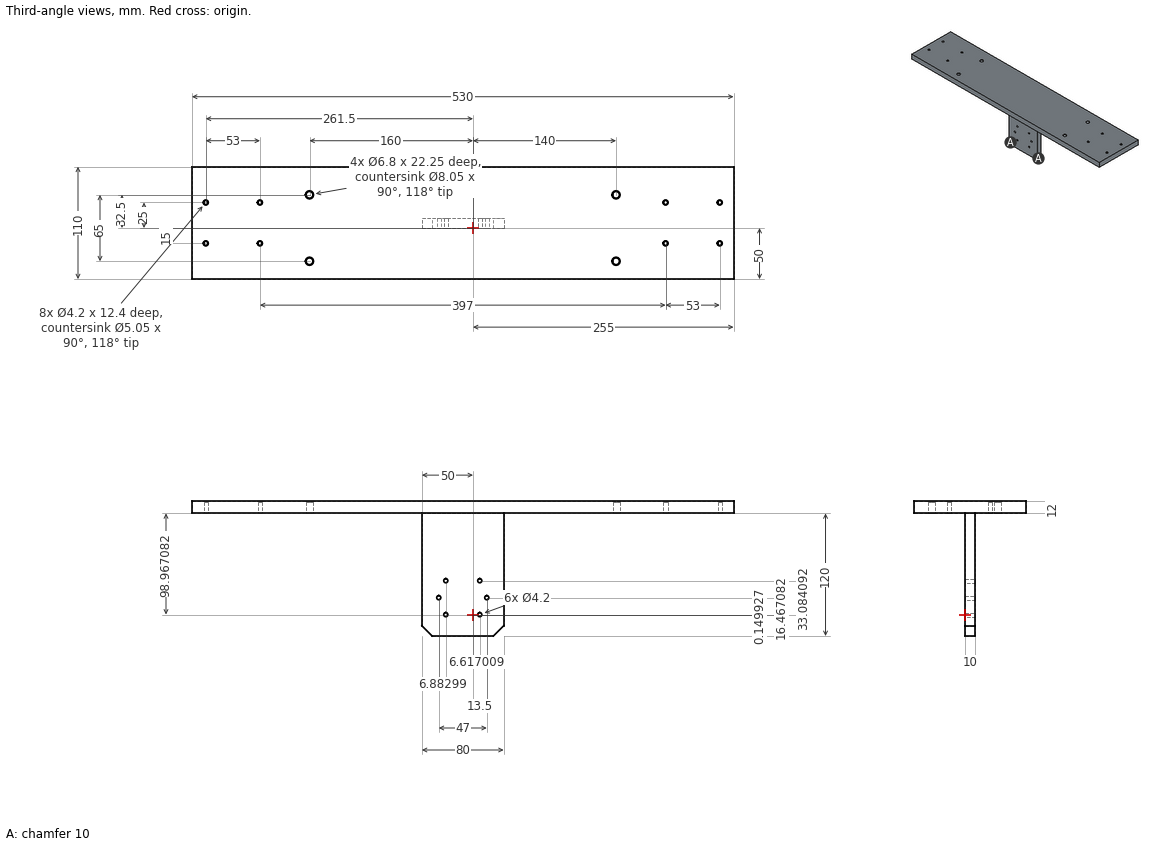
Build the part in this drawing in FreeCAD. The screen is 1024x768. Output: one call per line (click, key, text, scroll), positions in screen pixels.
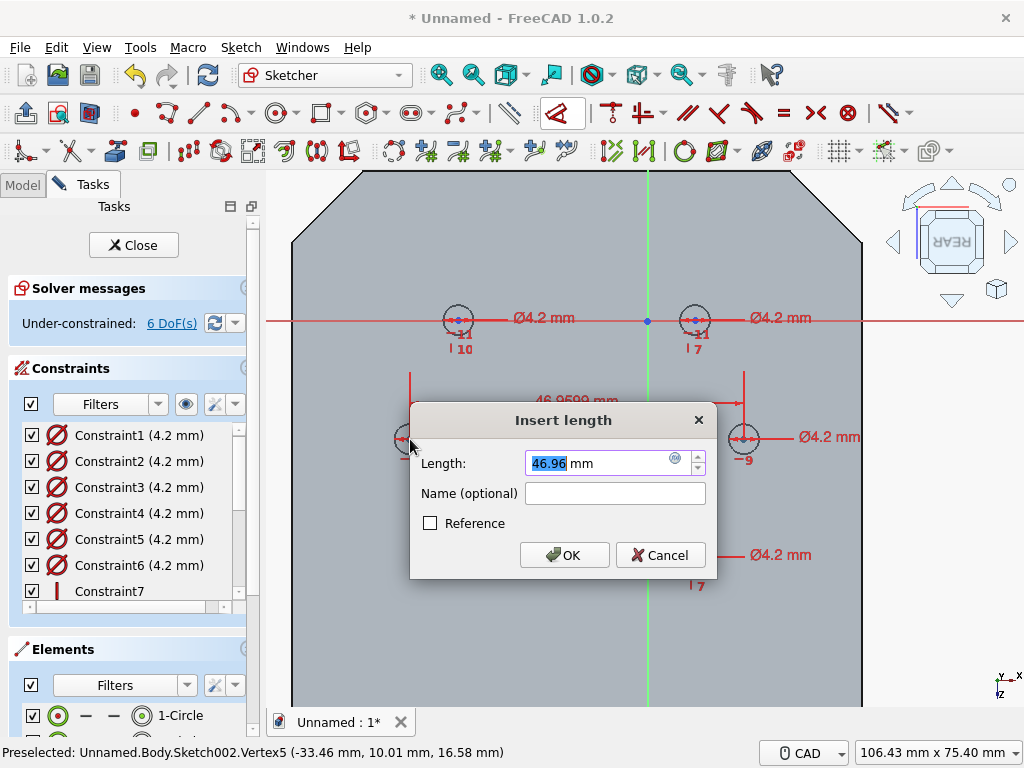
text(47)
key(Return)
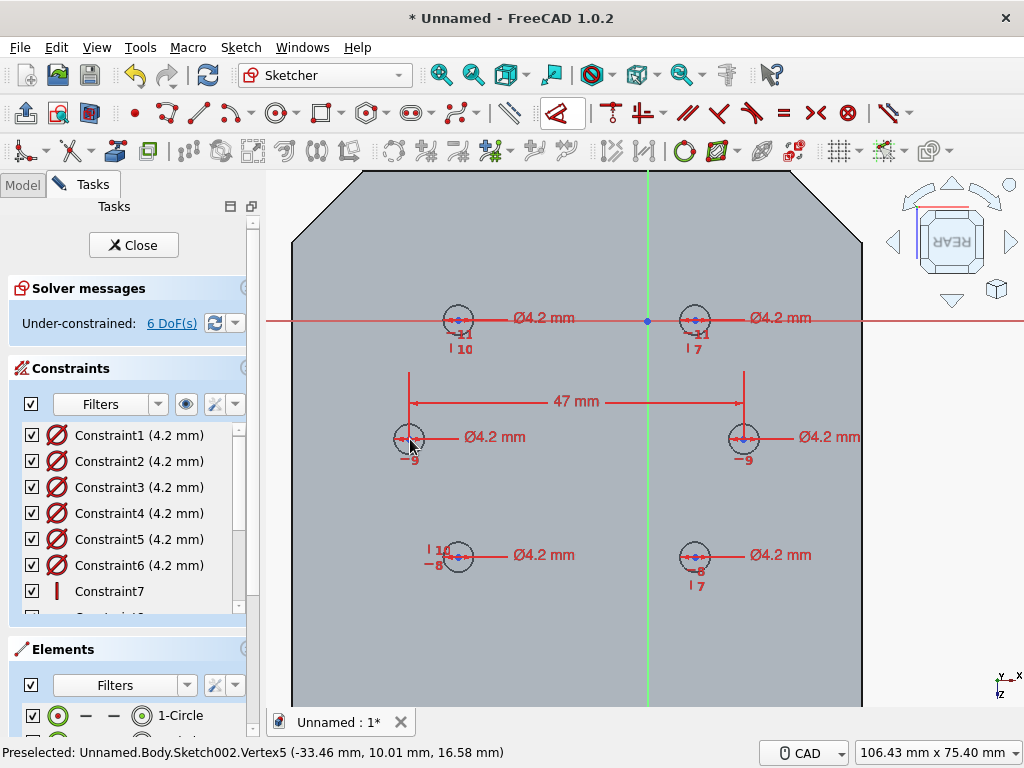
click(744, 439)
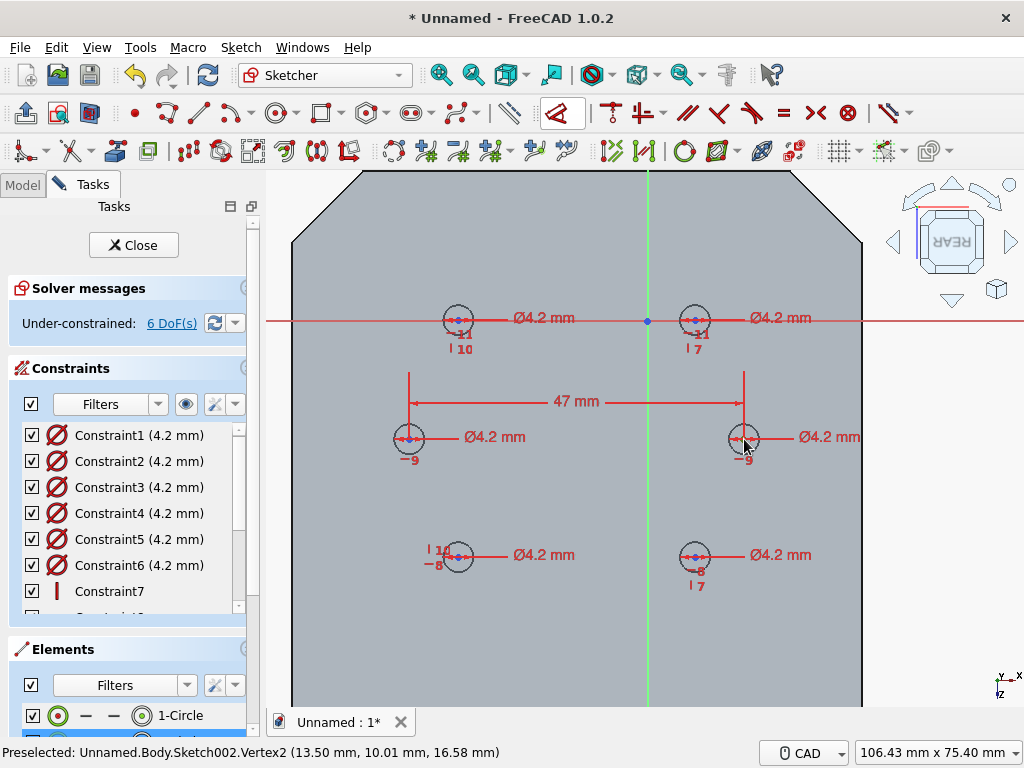
key(l)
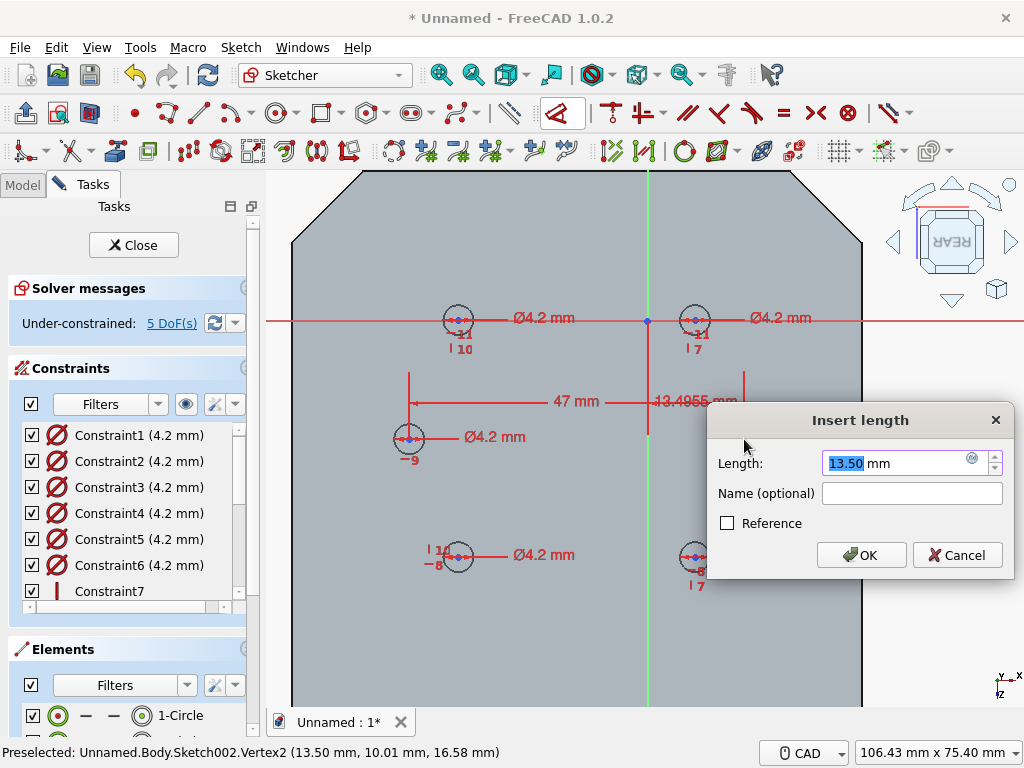
text(13.5)
key(Return)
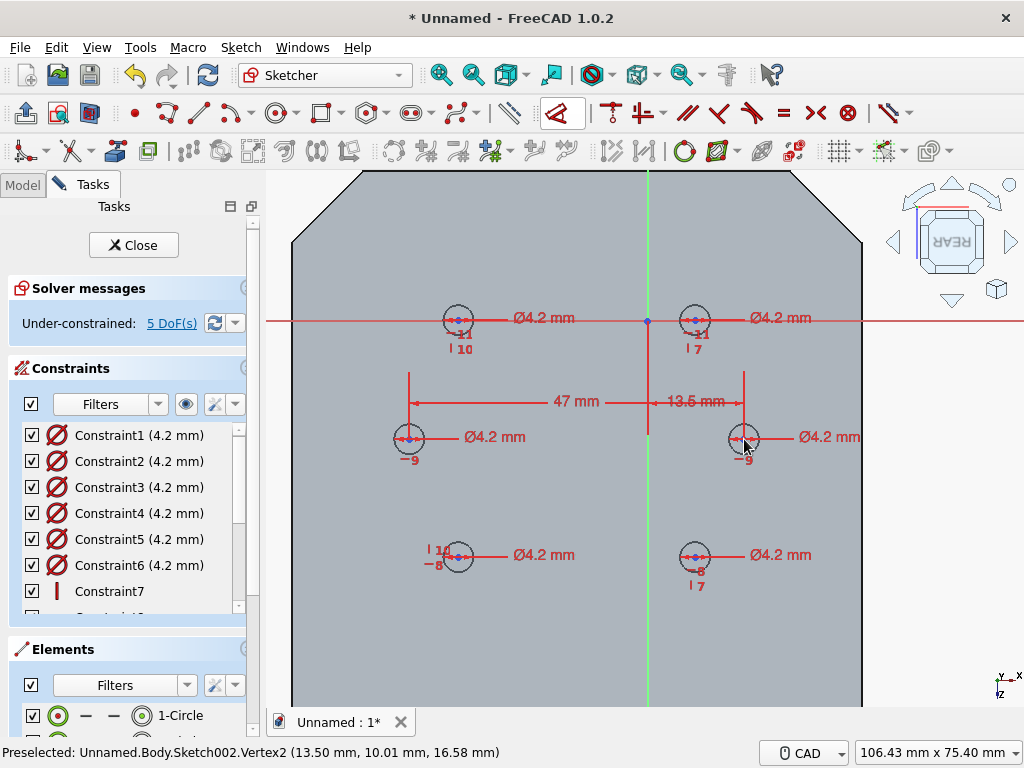
click(695, 320)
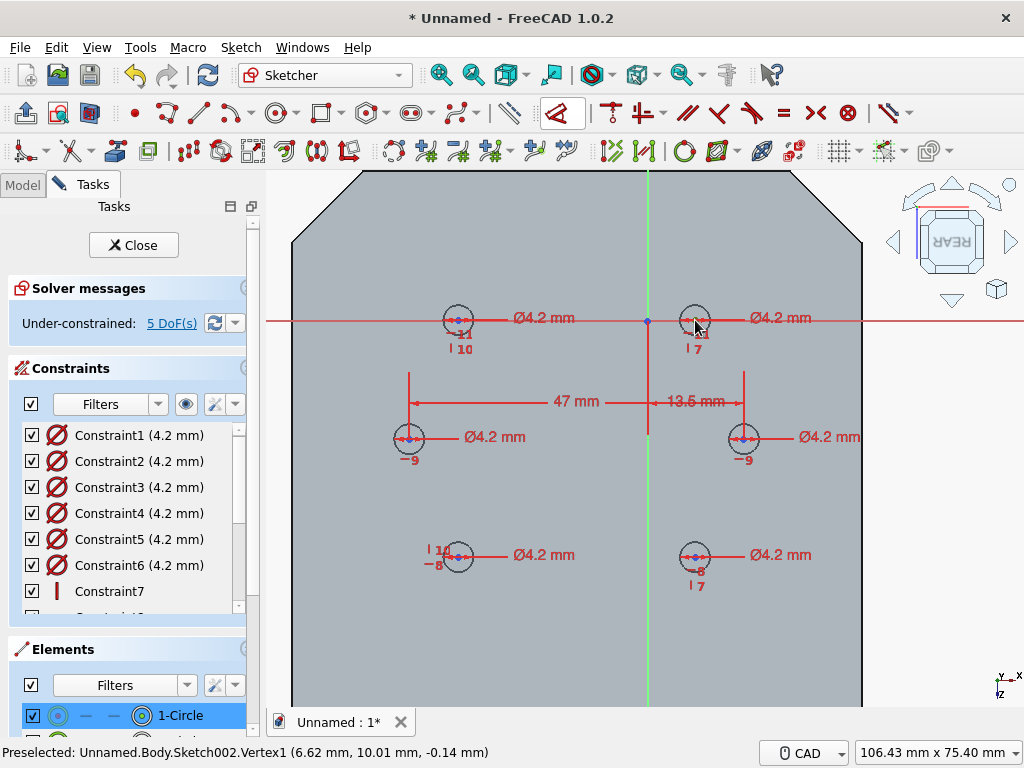
key(l)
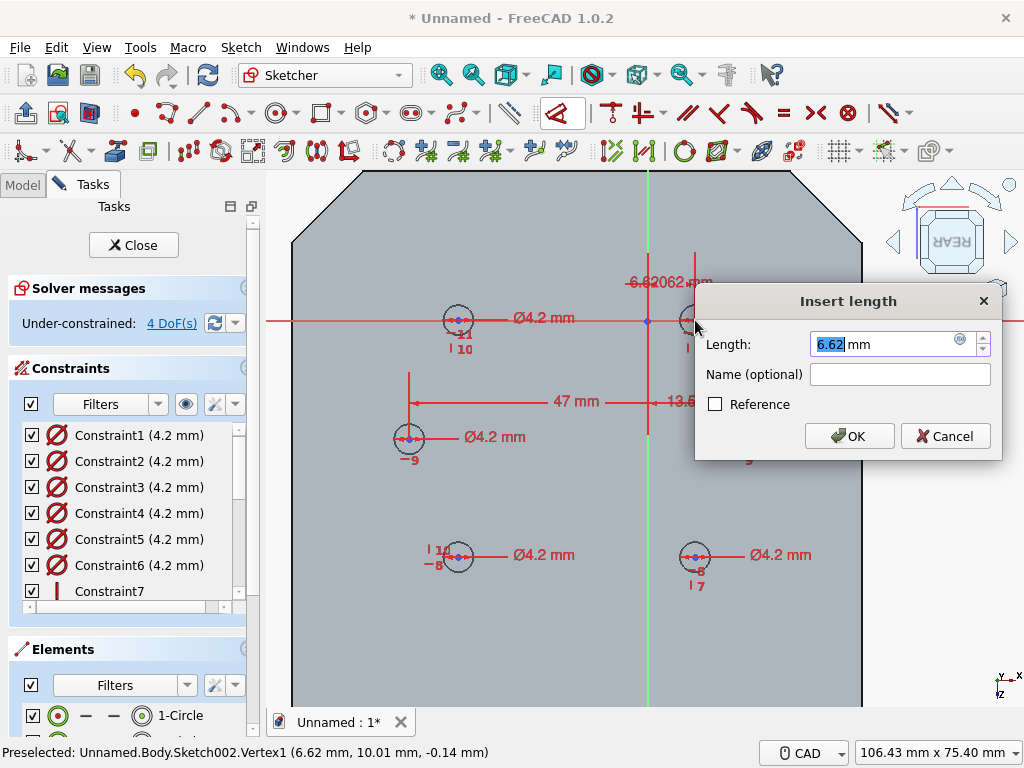
text(6.617009)
key(Return)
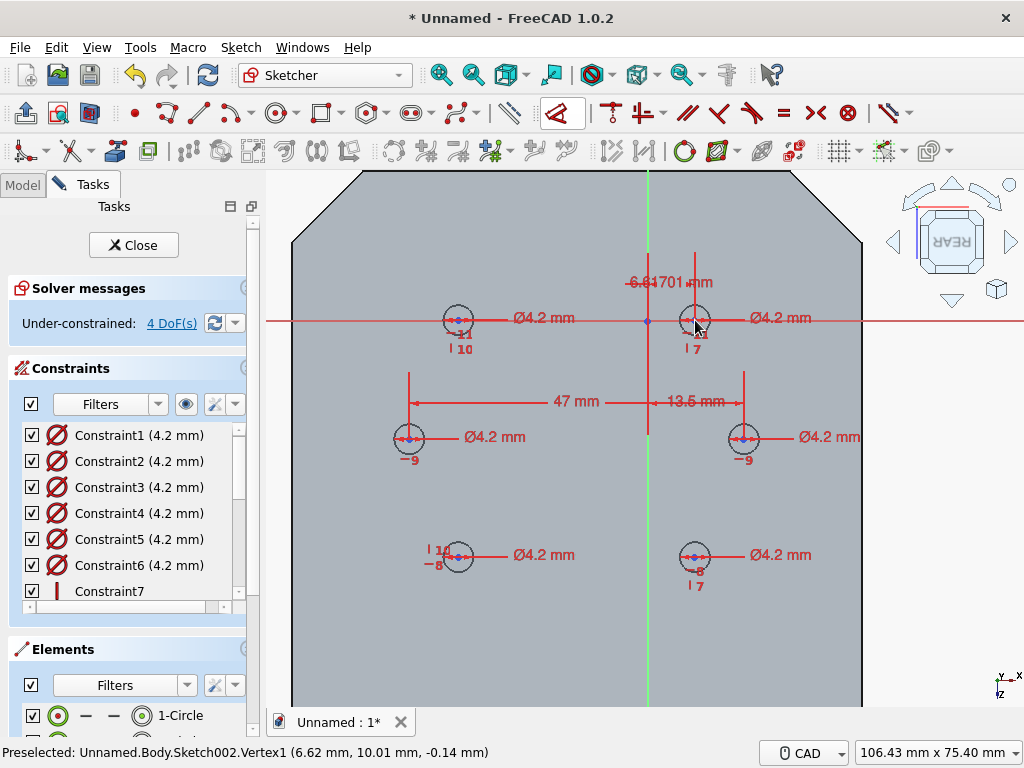
scroll(695, 320, up, 19)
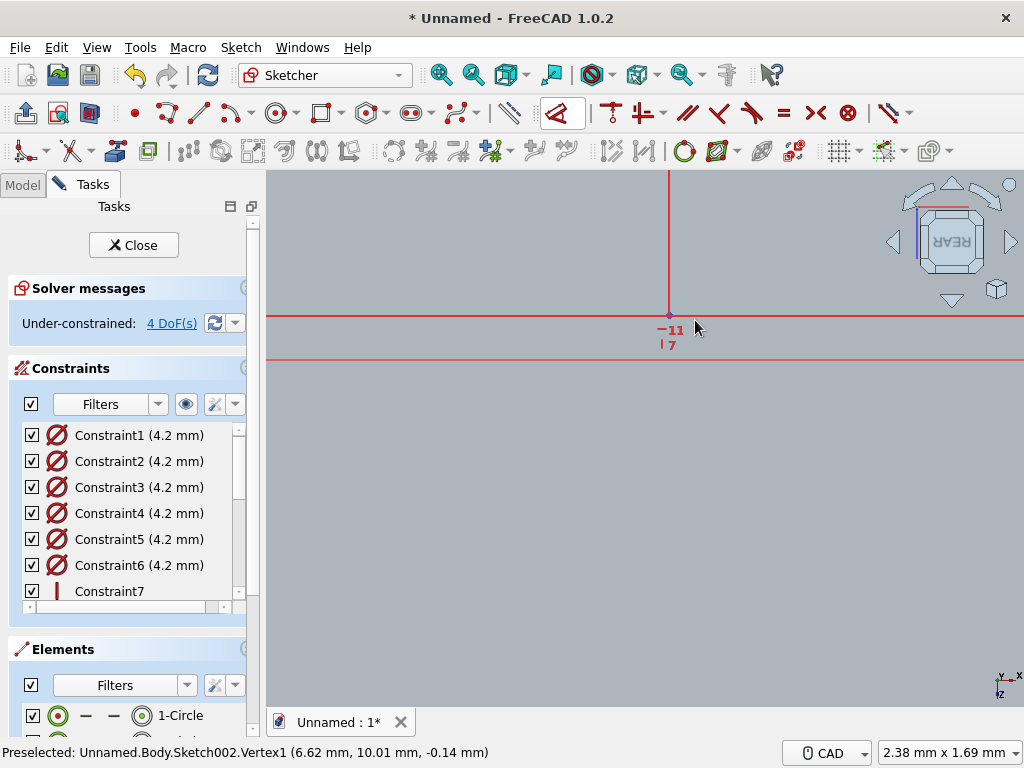
click(669, 316)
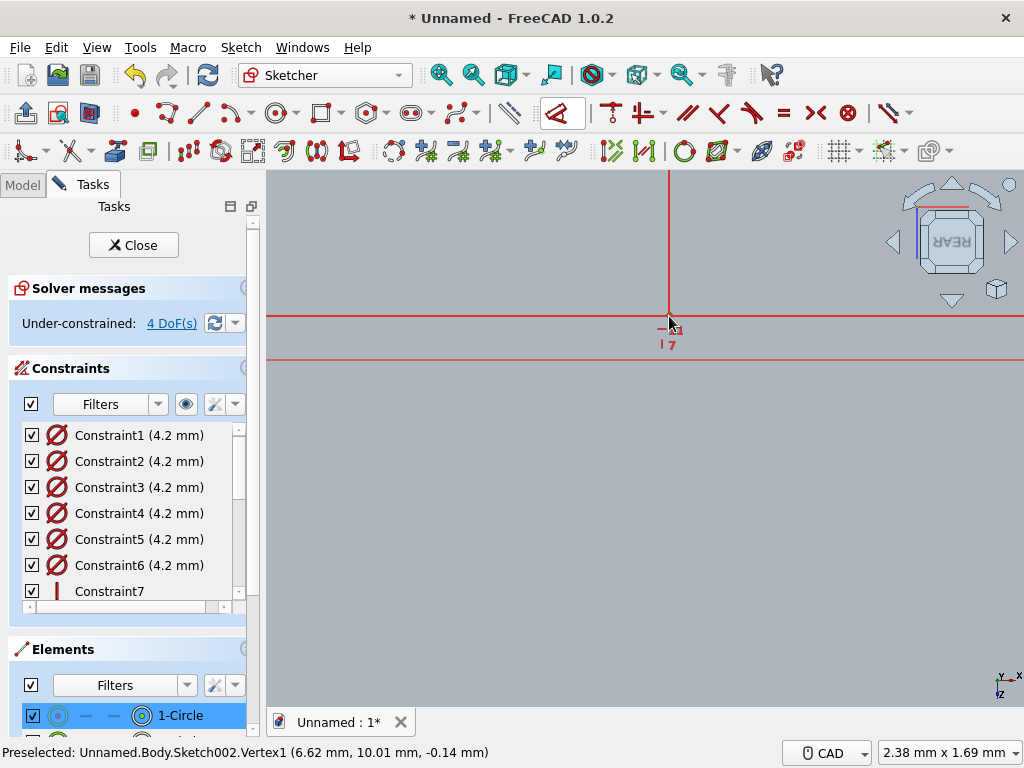
click(580, 114)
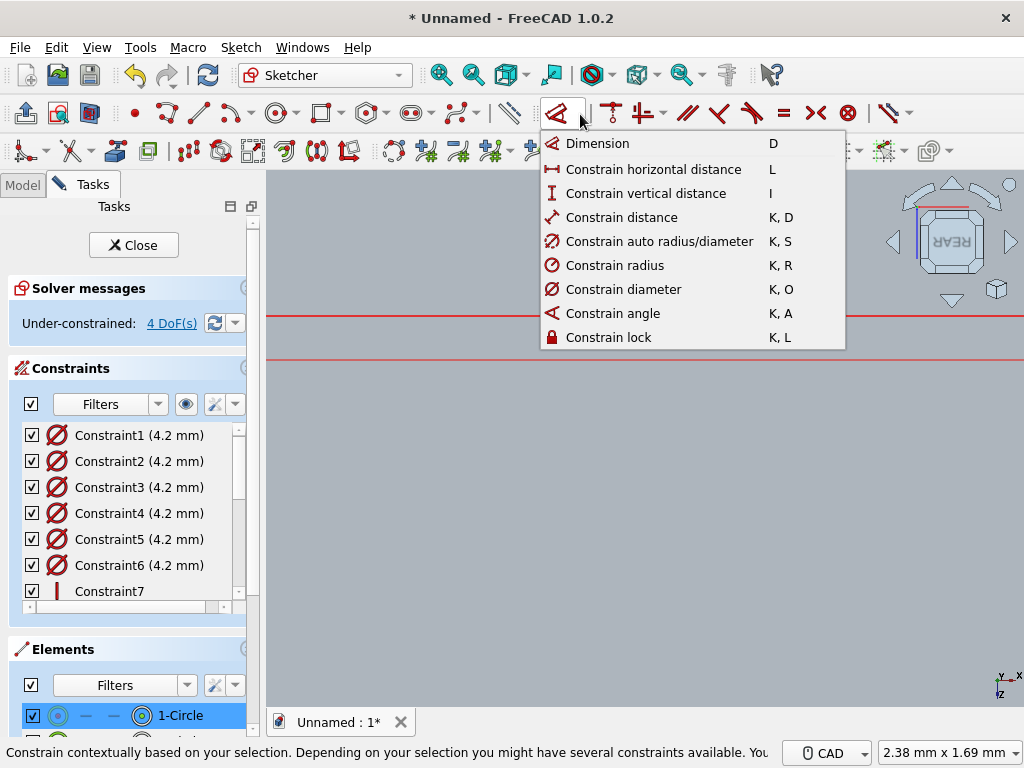
click(693, 193)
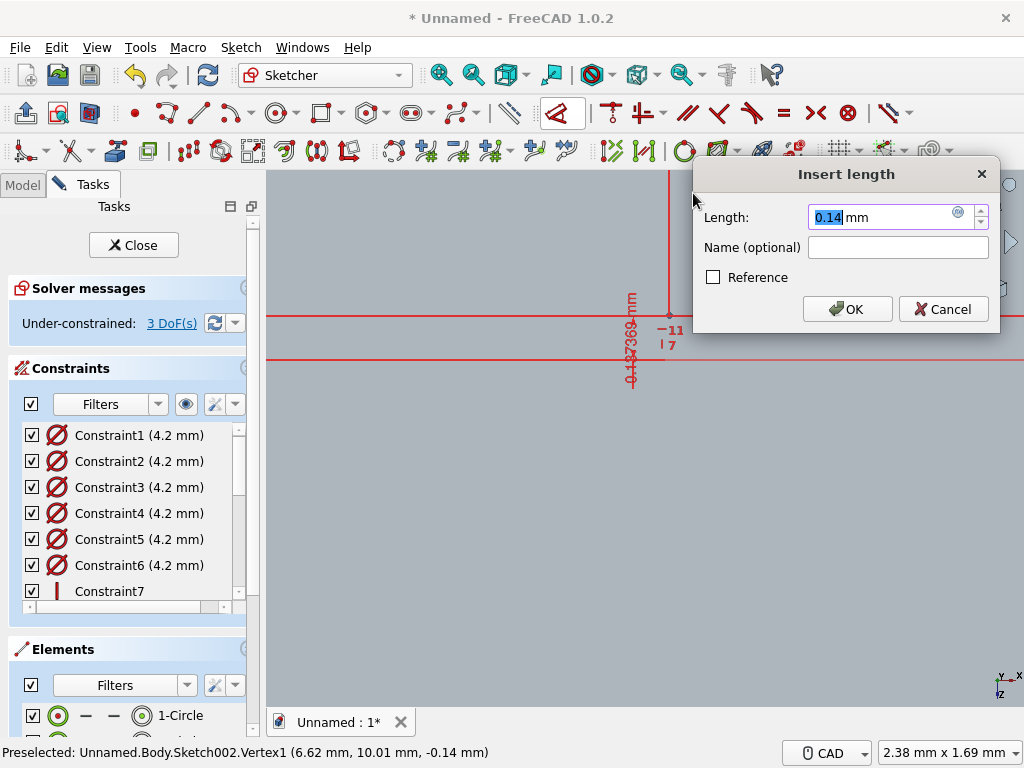
text(0.149927)
key(Return)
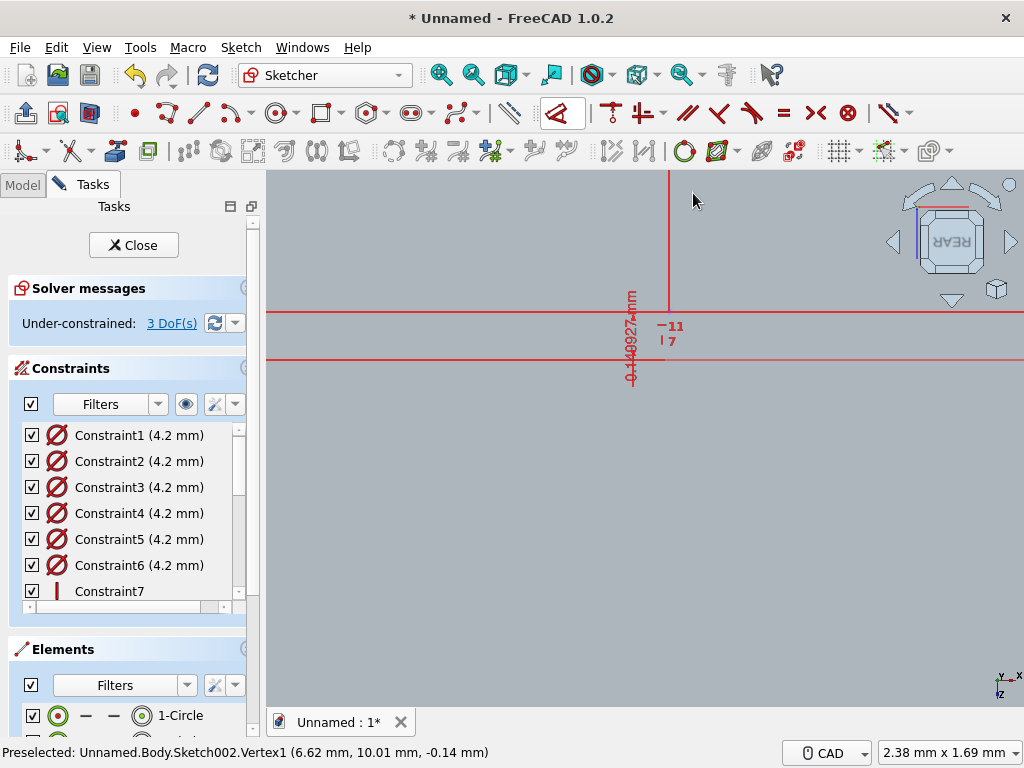
scroll(723, 293, down, 18)